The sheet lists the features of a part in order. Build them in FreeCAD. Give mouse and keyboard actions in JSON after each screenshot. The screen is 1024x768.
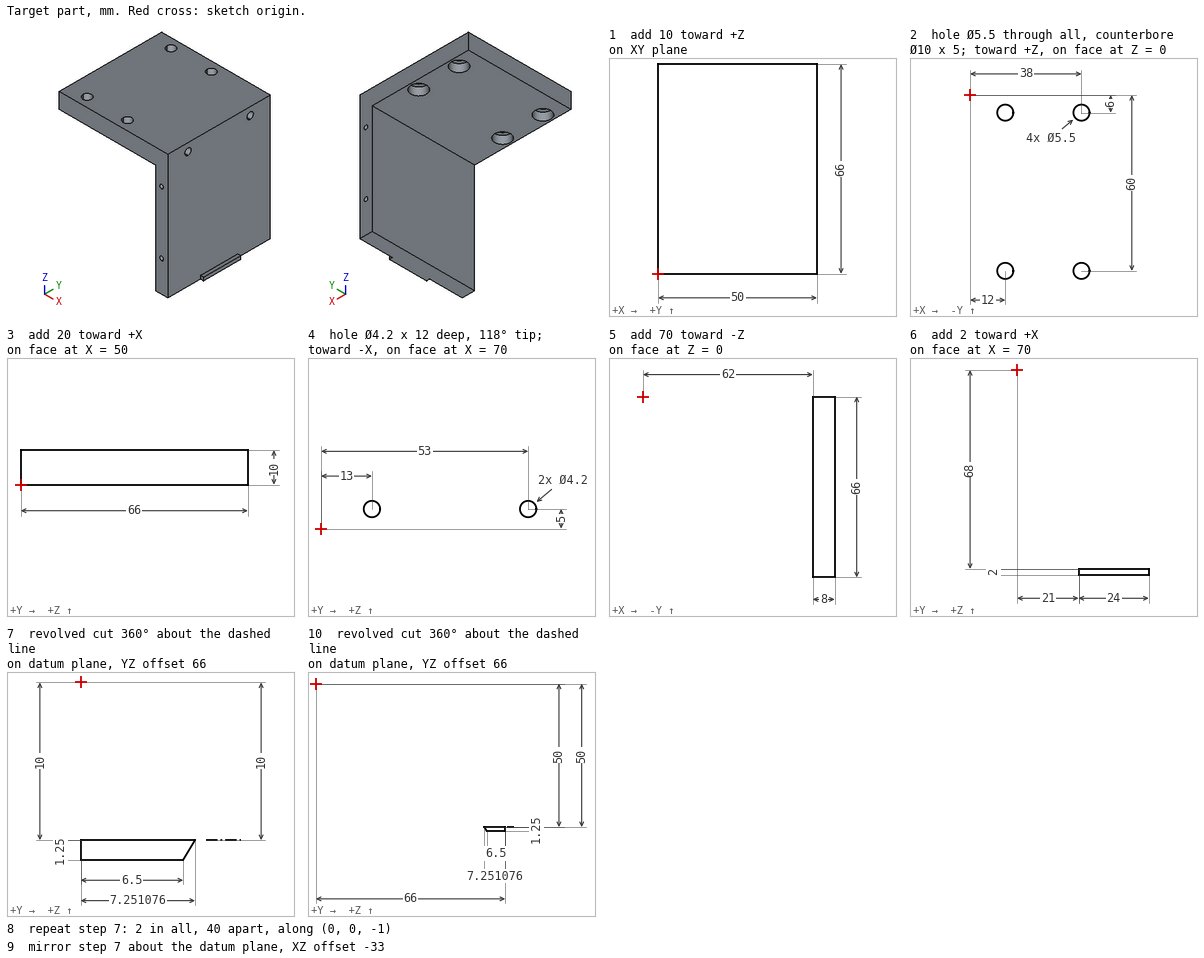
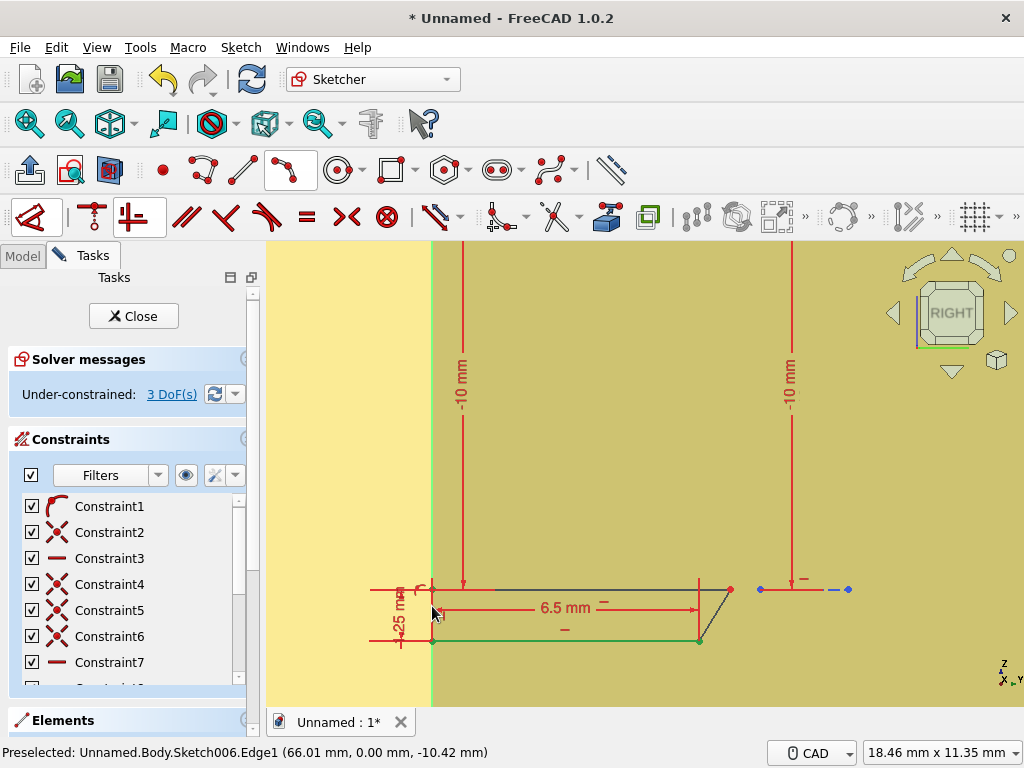
{"action": "left_click", "coordinate": [641, 590]}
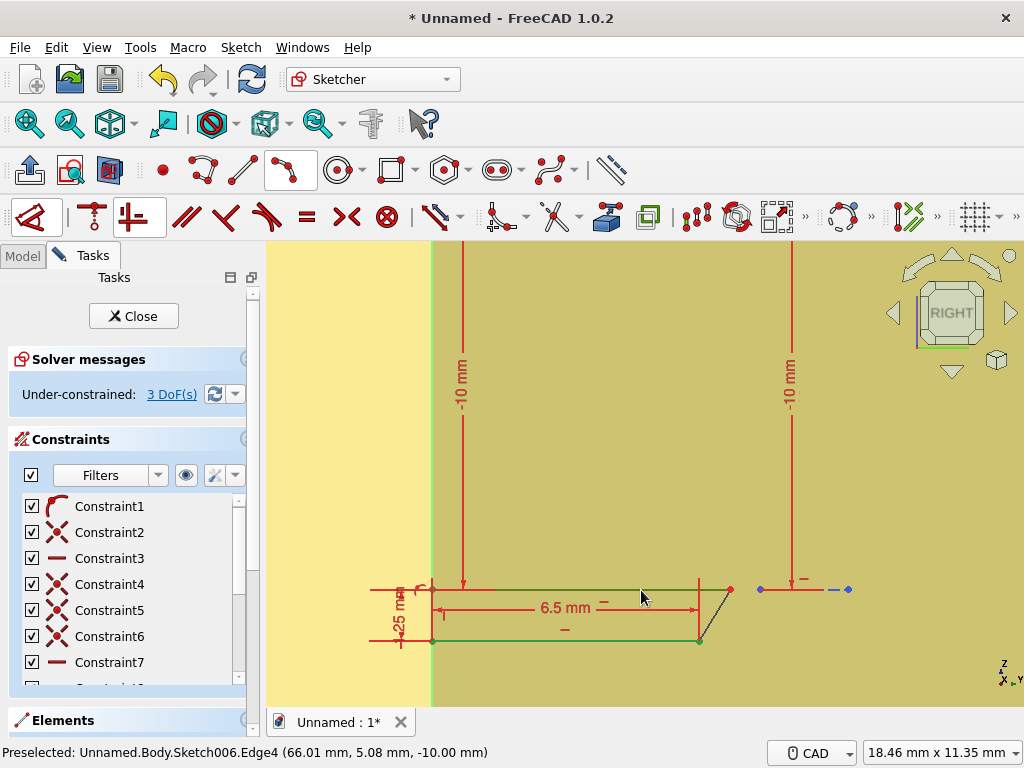
{"action": "key", "text": "l"}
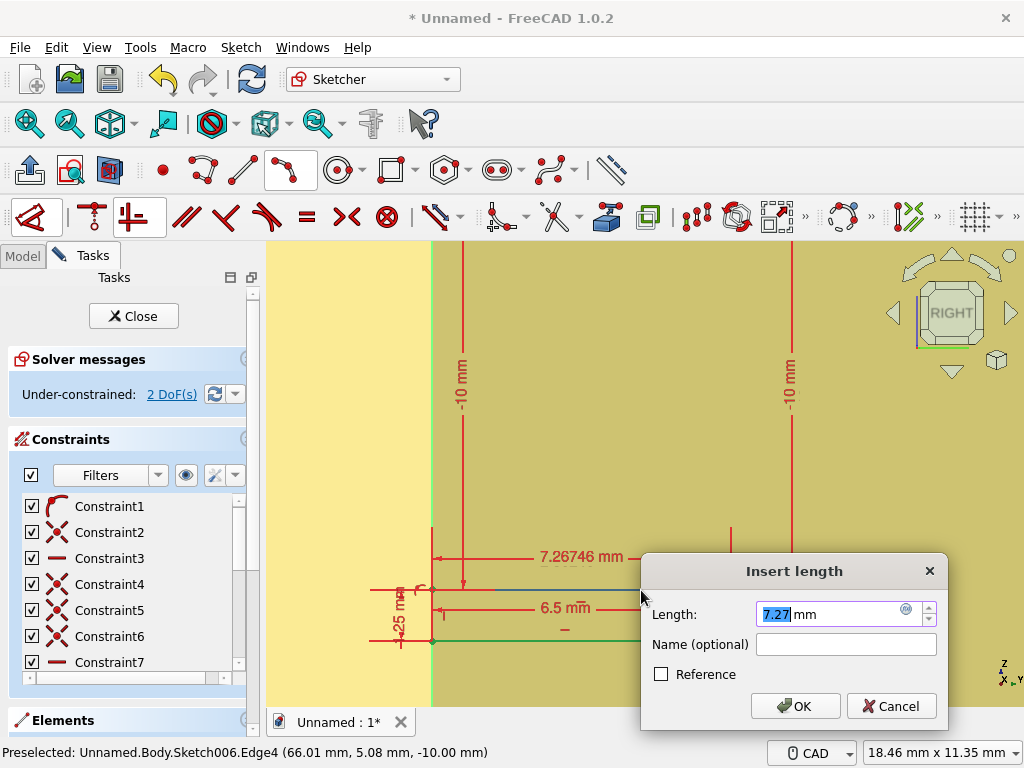
{"action": "type", "text": "7.251076"}
{"action": "key", "text": "Return"}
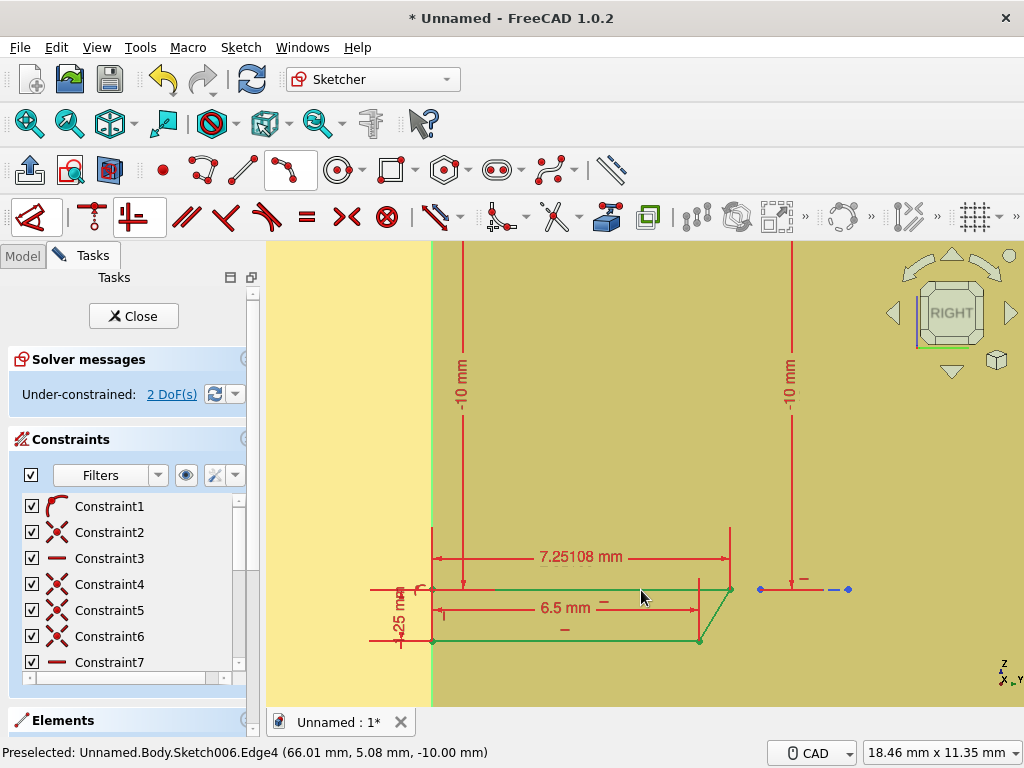
{"action": "left_click", "coordinate": [134, 316]}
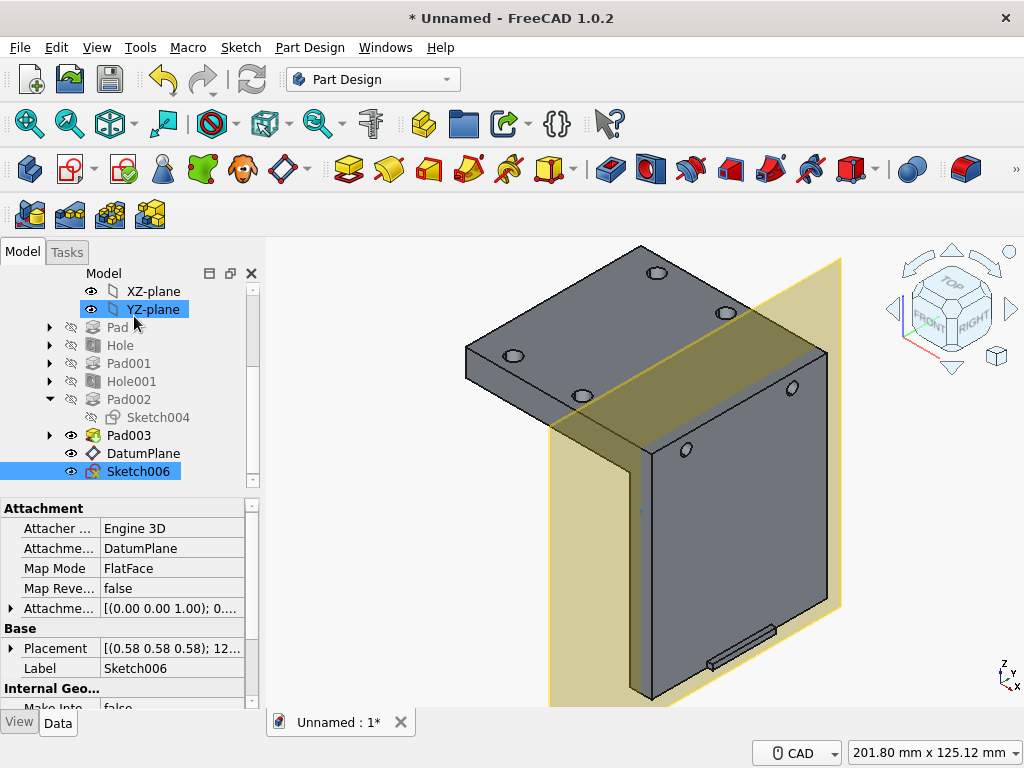
{"action": "left_click", "coordinate": [692, 170]}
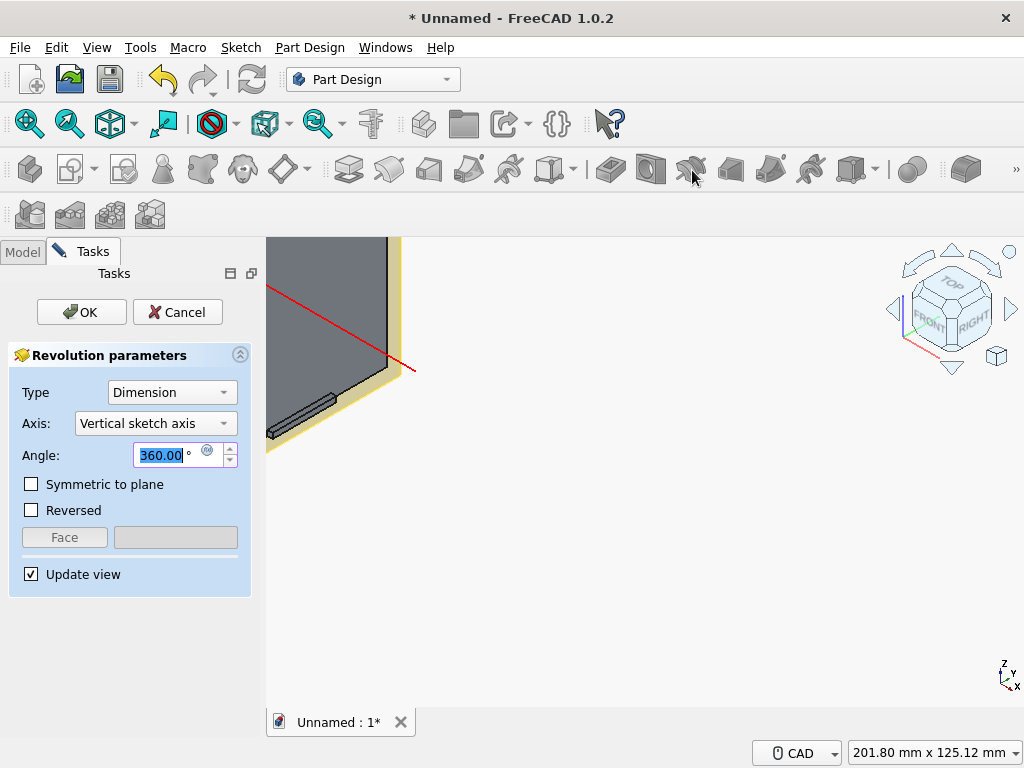
{"action": "left_click", "coordinate": [156, 424]}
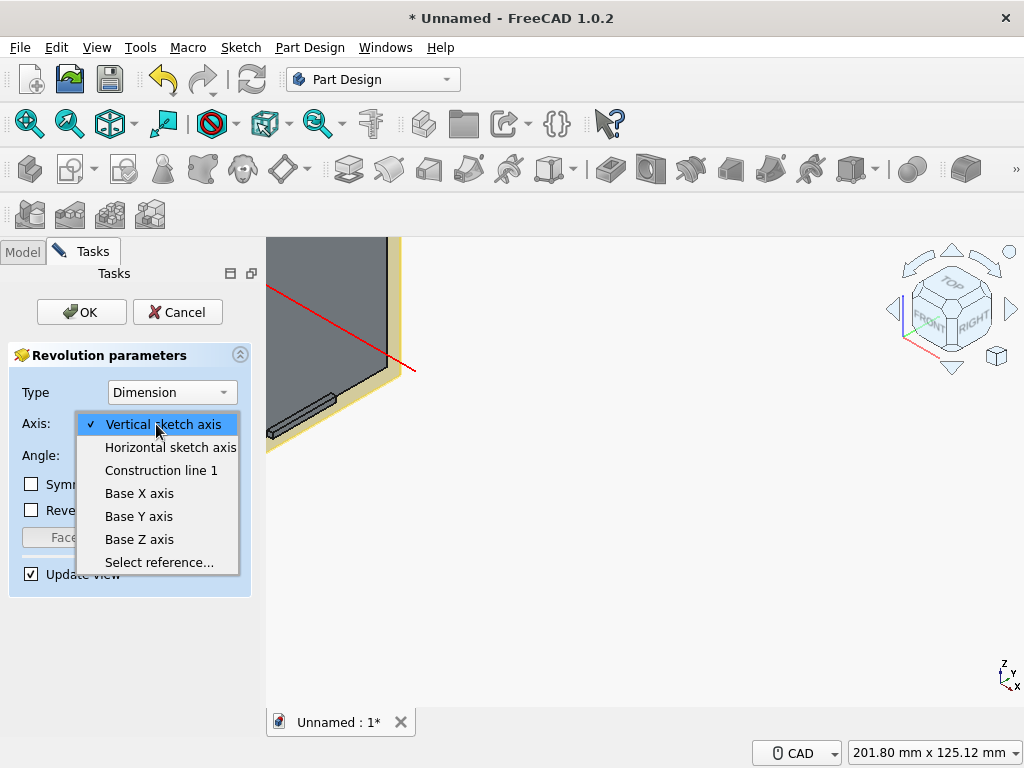
{"action": "left_click", "coordinate": [156, 470]}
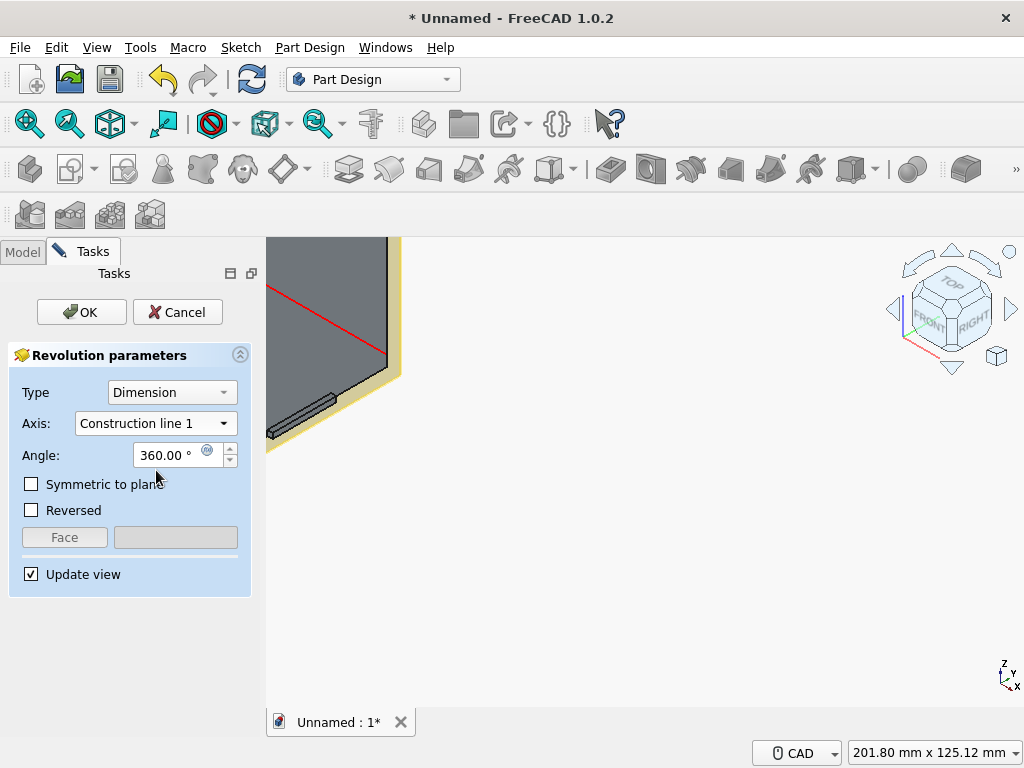
{"action": "left_click", "coordinate": [82, 312]}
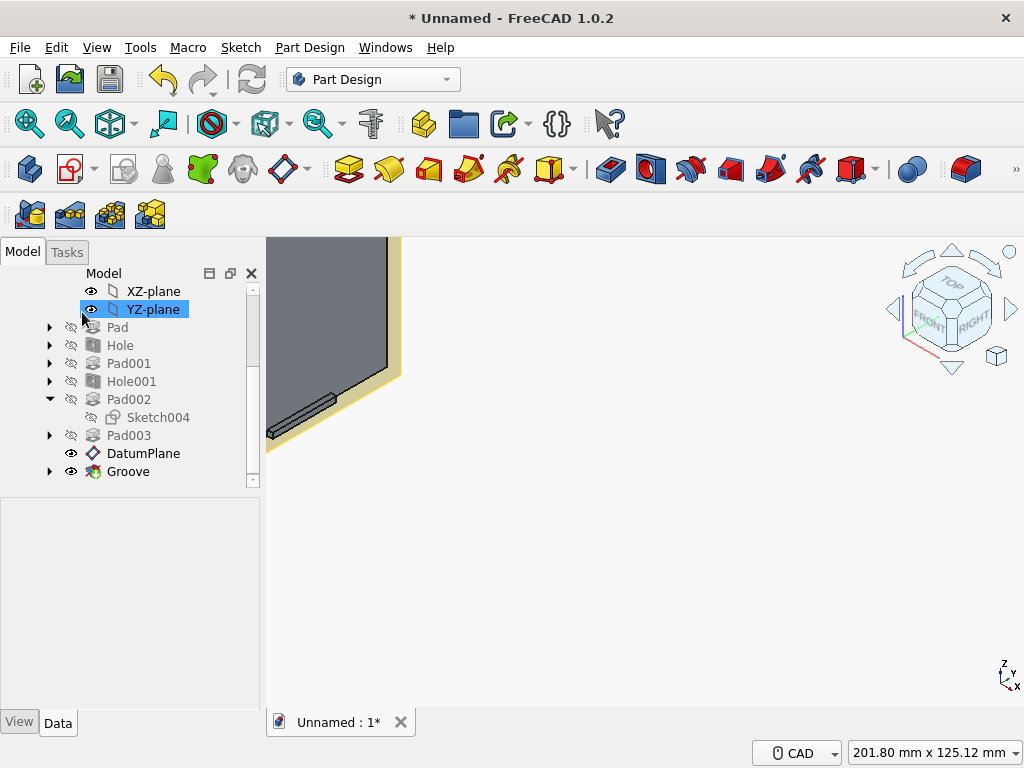
{"action": "left_click", "coordinate": [116, 453]}
{"action": "key", "text": "space"}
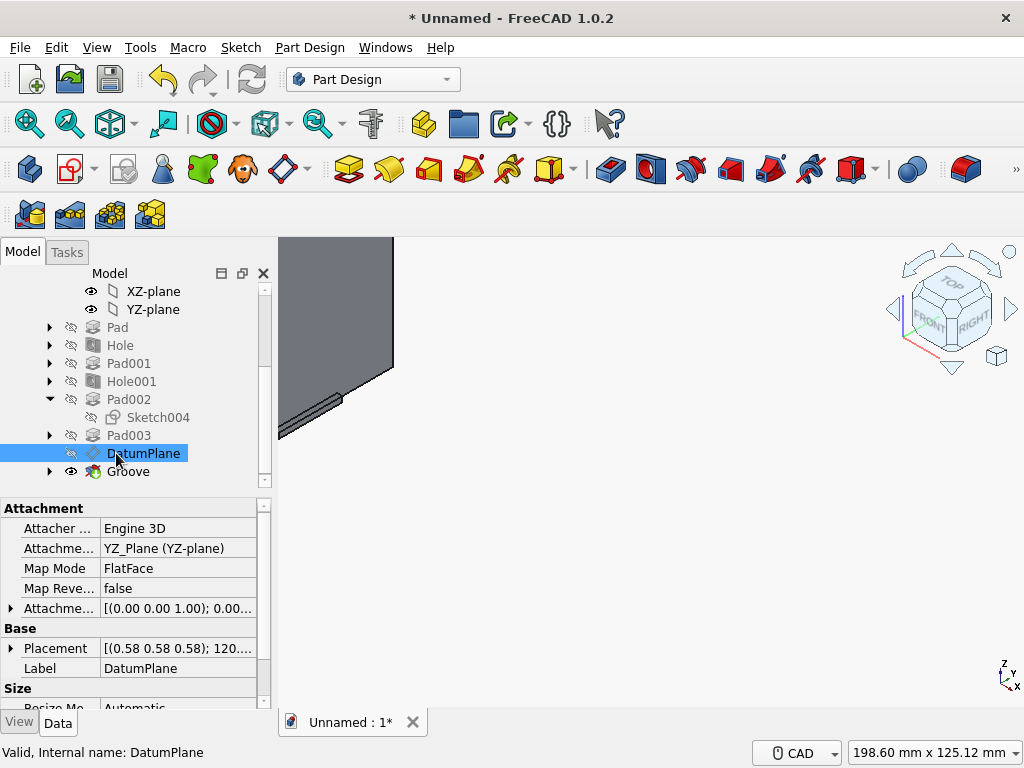
{"action": "left_click", "coordinate": [30, 124]}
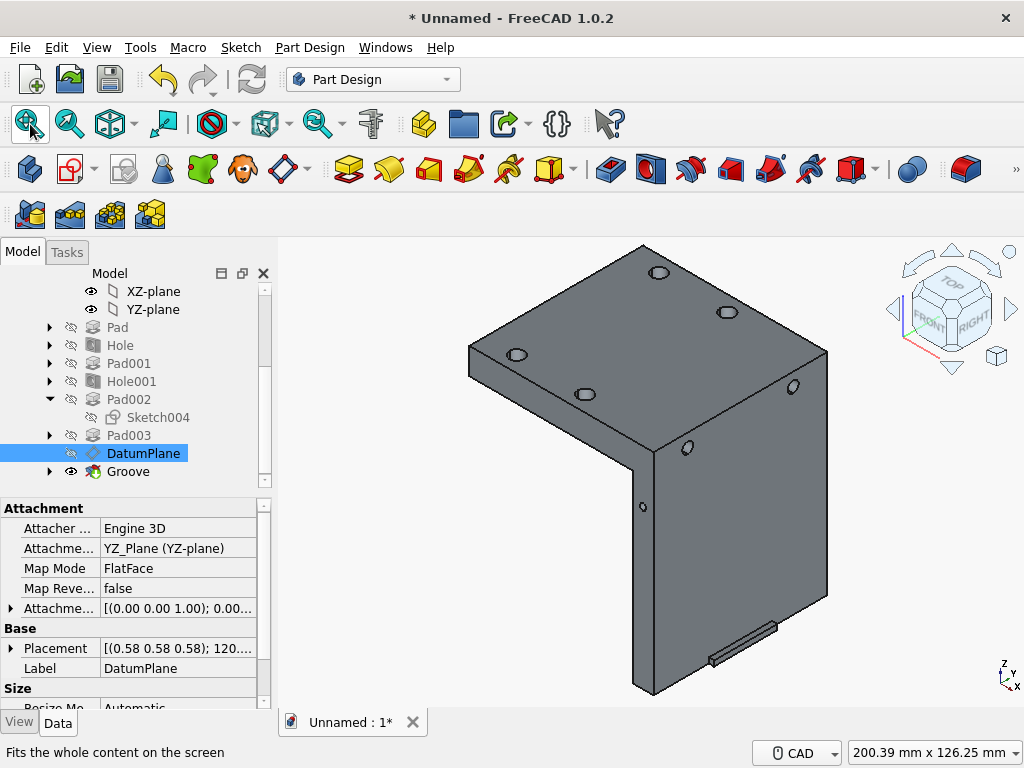
{"action": "left_click", "coordinate": [116, 471]}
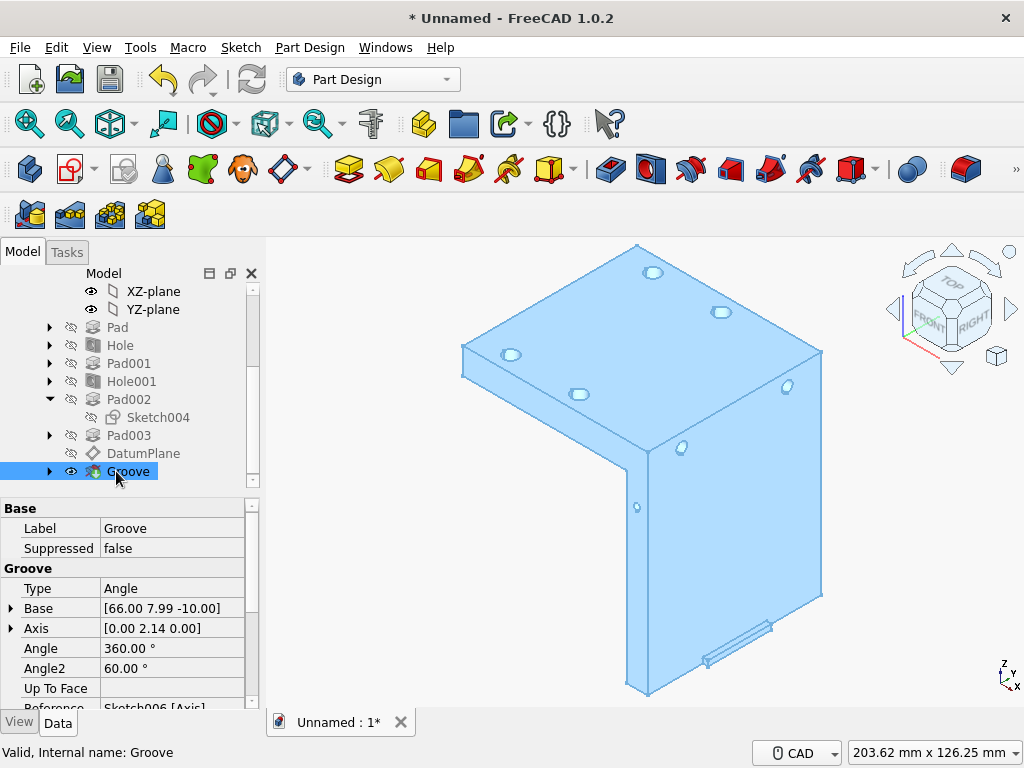
{"action": "left_click", "coordinate": [70, 214]}